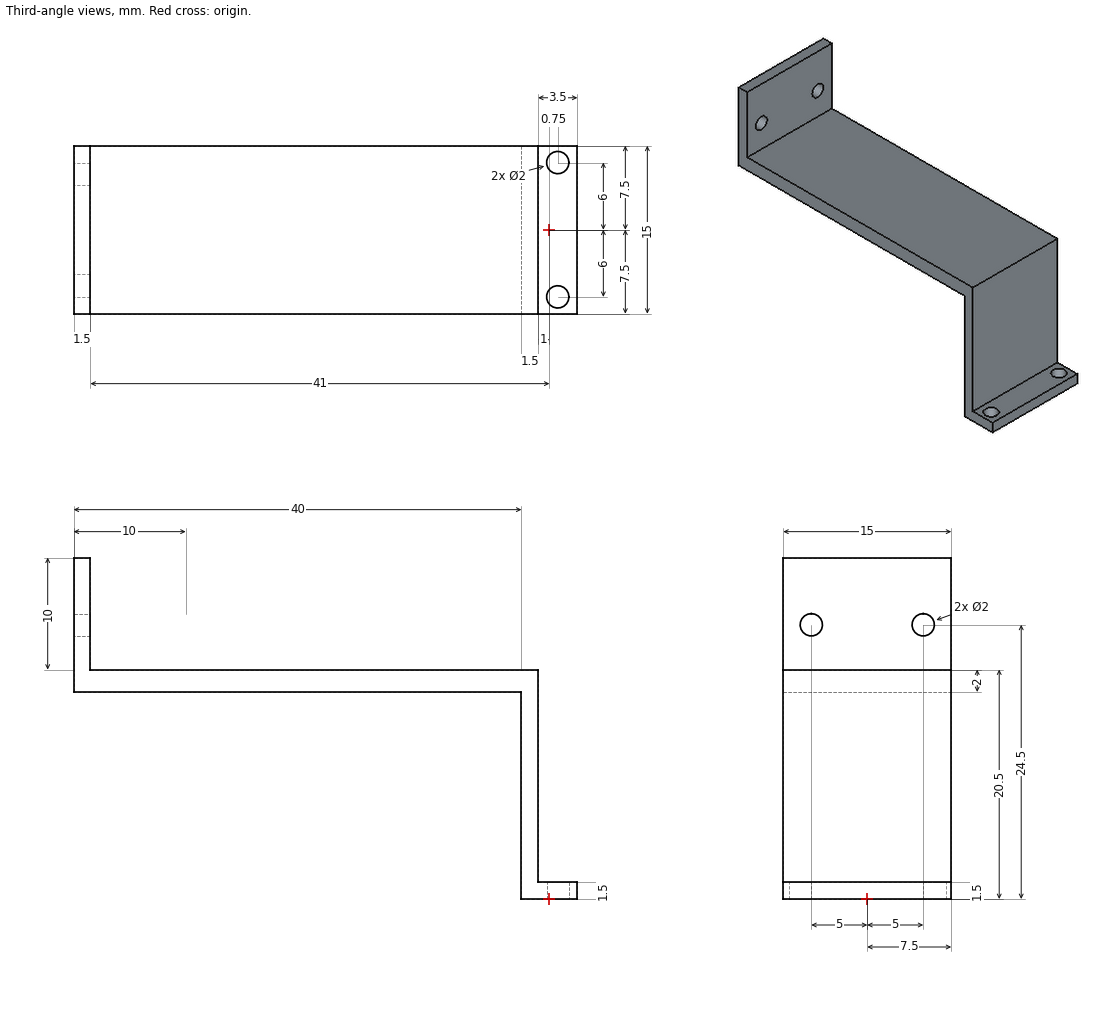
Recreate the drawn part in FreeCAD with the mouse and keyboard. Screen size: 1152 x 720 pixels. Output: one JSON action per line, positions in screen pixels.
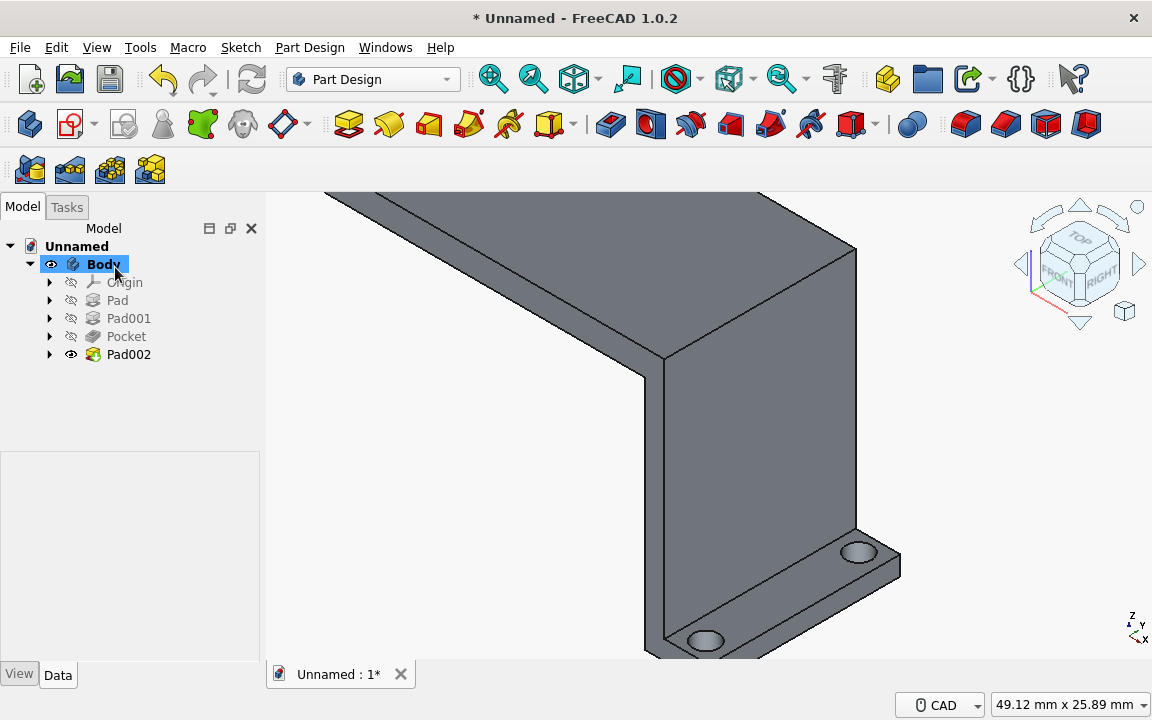
{"action": "left_click", "coordinate": [494, 80]}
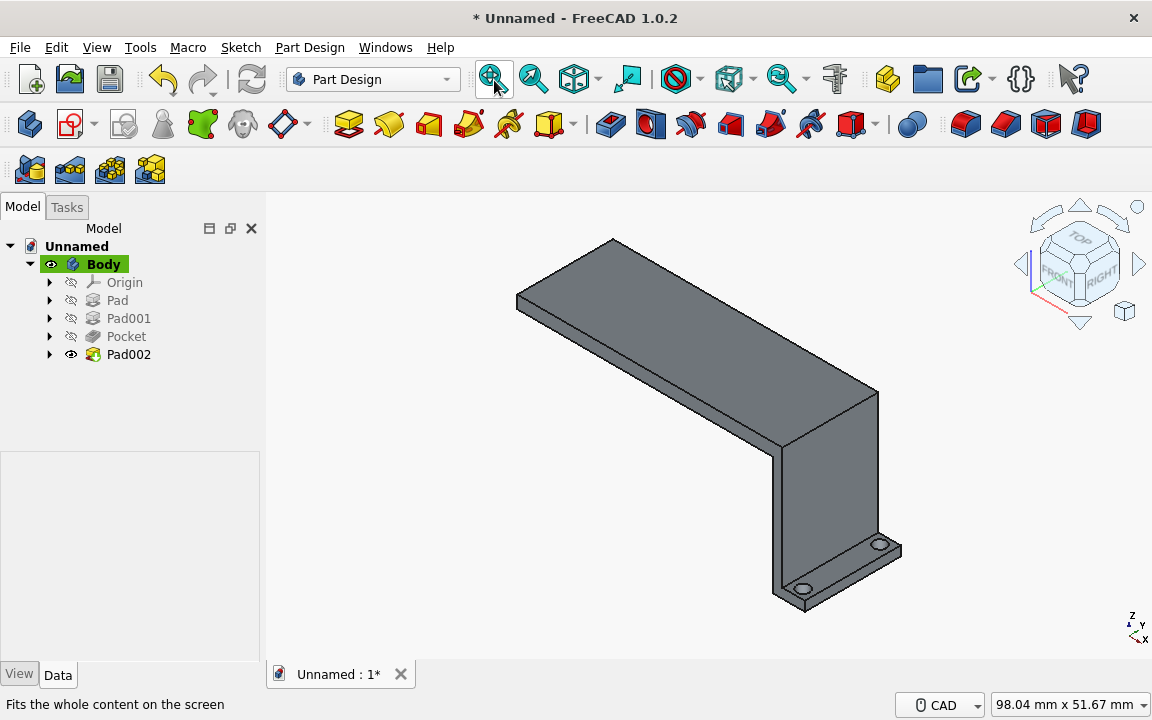
{"action": "left_click", "coordinate": [774, 386]}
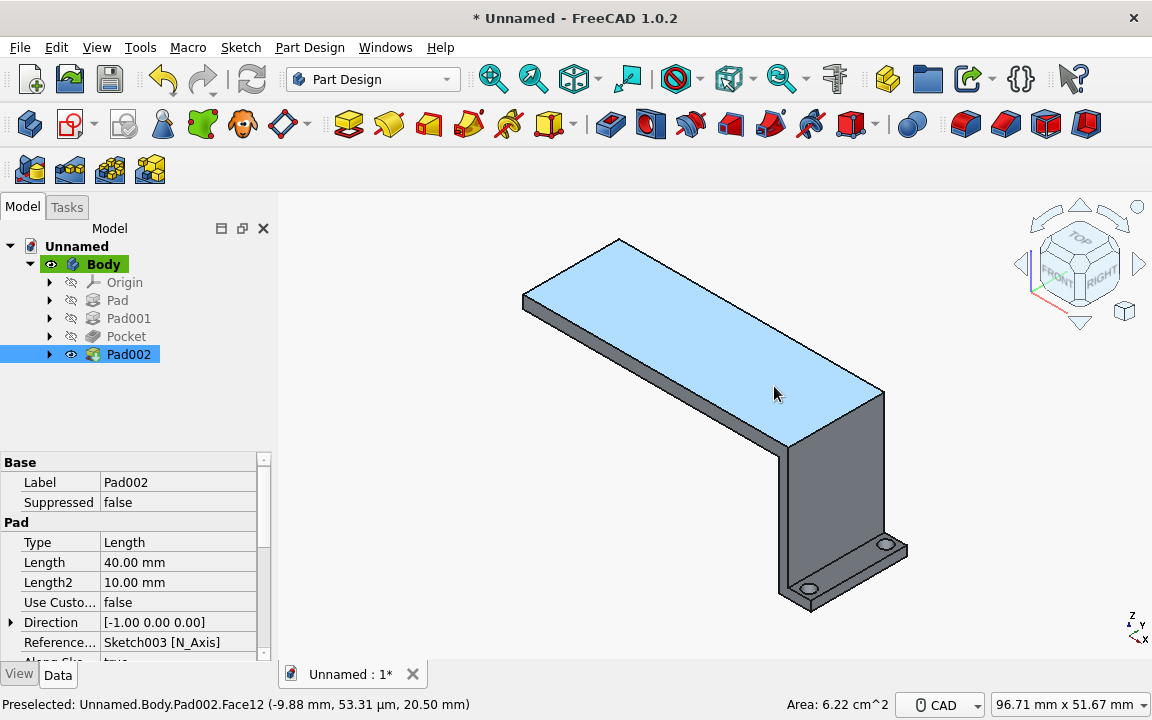
{"action": "left_click", "coordinate": [70, 124]}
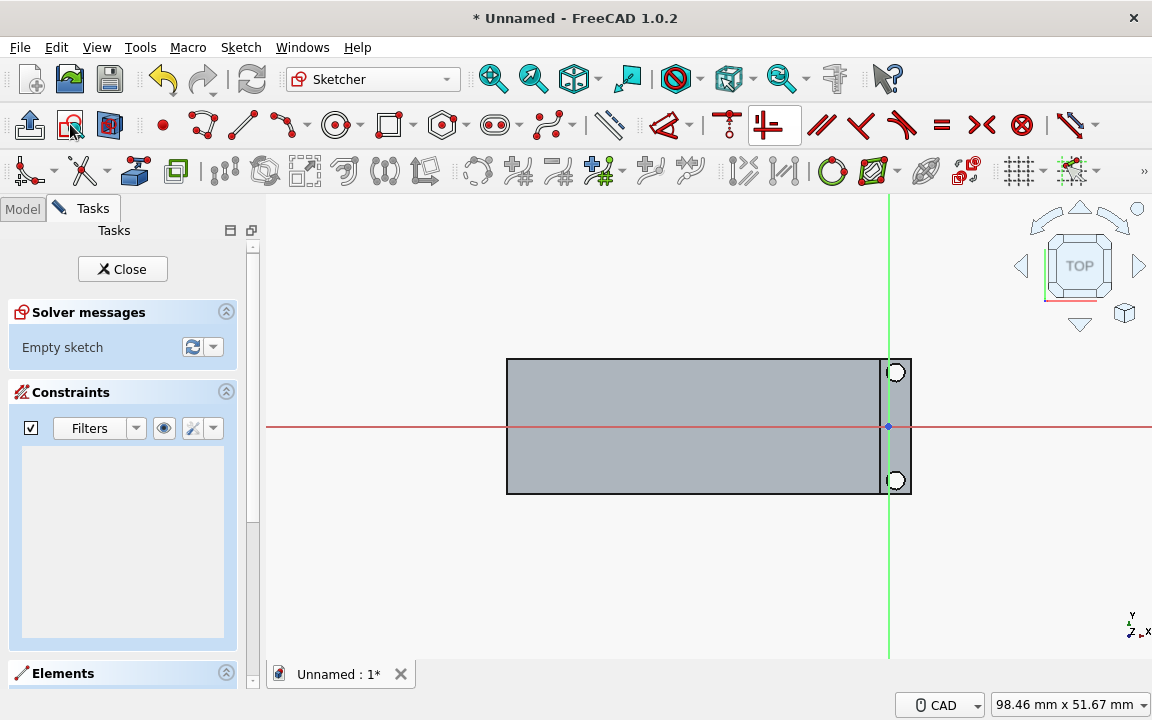
{"action": "scroll", "coordinate": [409, 426], "scroll_direction": "up", "scroll_amount": 4}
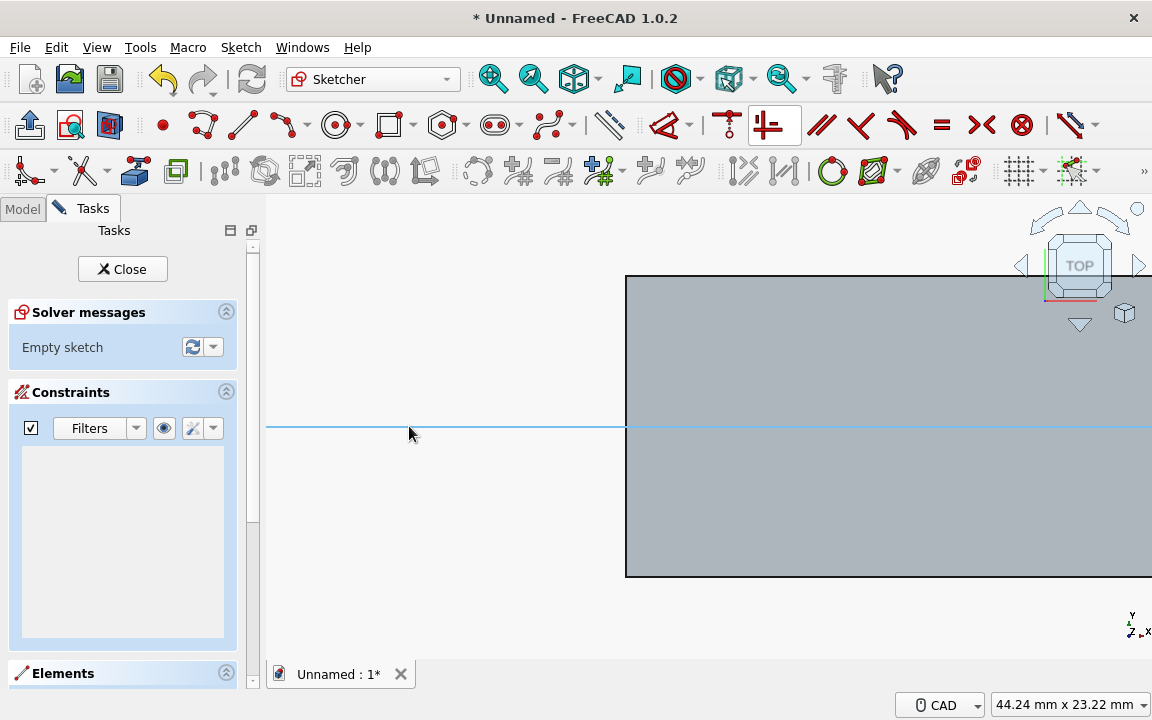
{"action": "left_click", "coordinate": [390, 126]}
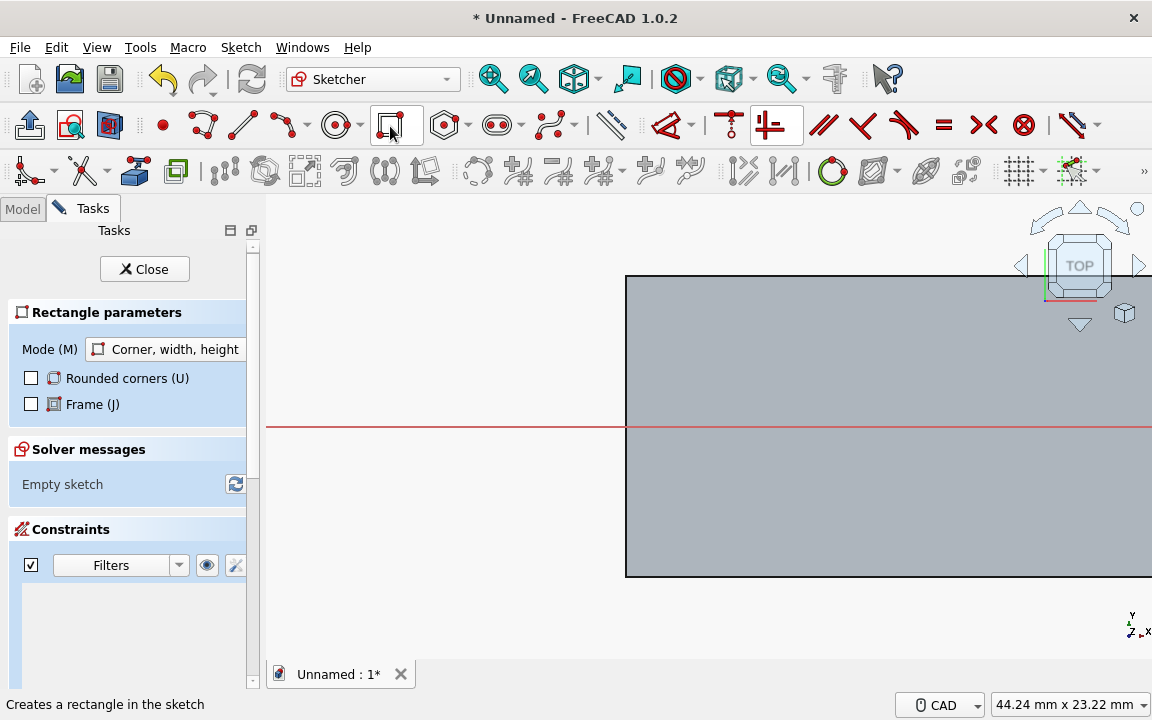
{"action": "left_click", "coordinate": [626, 276]}
{"action": "left_click", "coordinate": [656, 577]}
{"action": "key", "text": "Escape"}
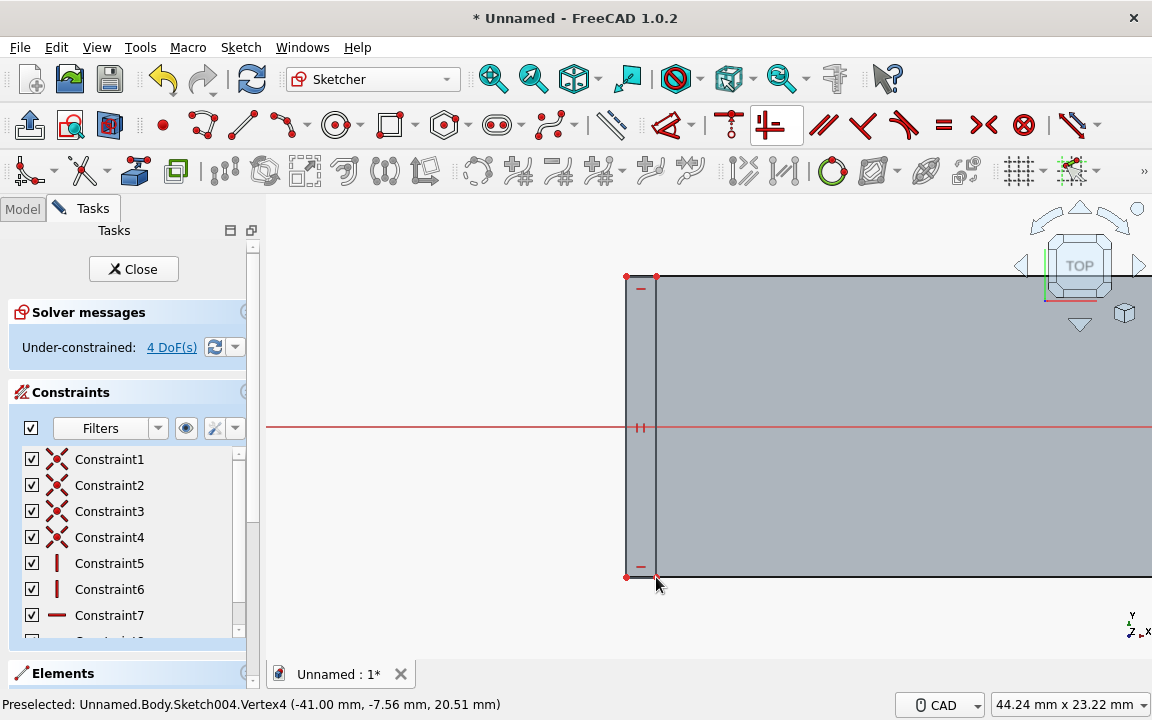
{"action": "left_click", "coordinate": [666, 126]}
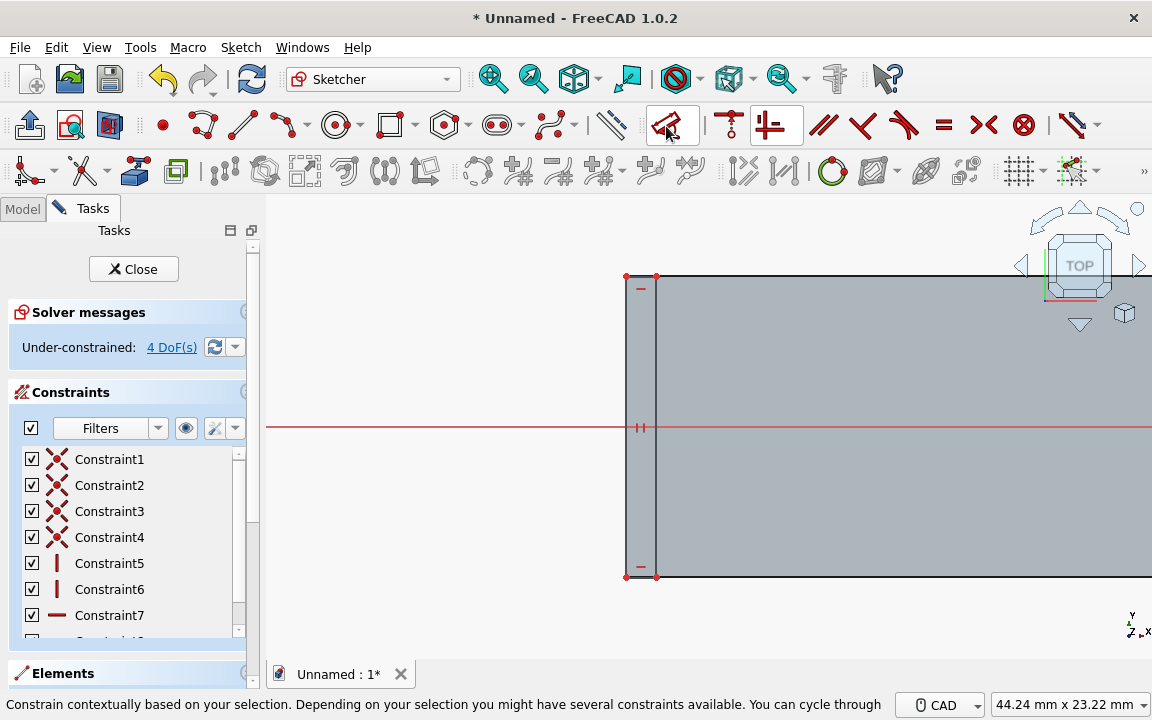
{"action": "left_click", "coordinate": [626, 367]}
{"action": "left_click", "coordinate": [592, 358]}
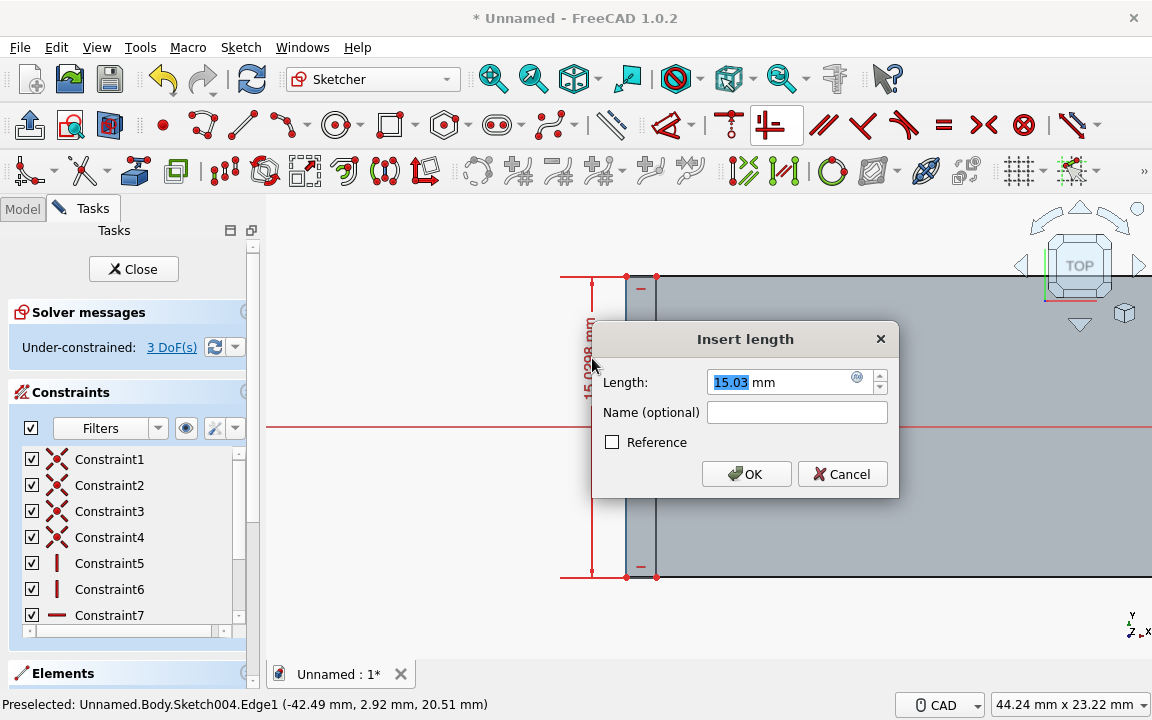
{"action": "type", "text": "15"}
{"action": "key", "text": "Return"}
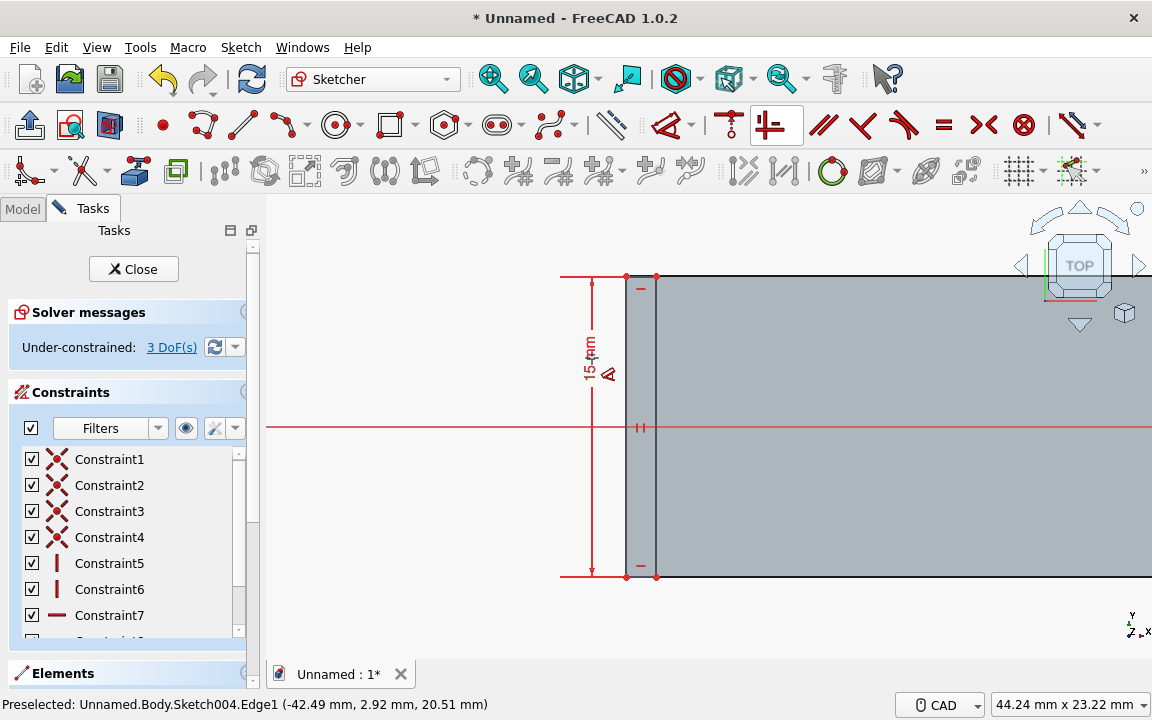
{"action": "scroll", "coordinate": [638, 577], "scroll_direction": "up", "scroll_amount": 2}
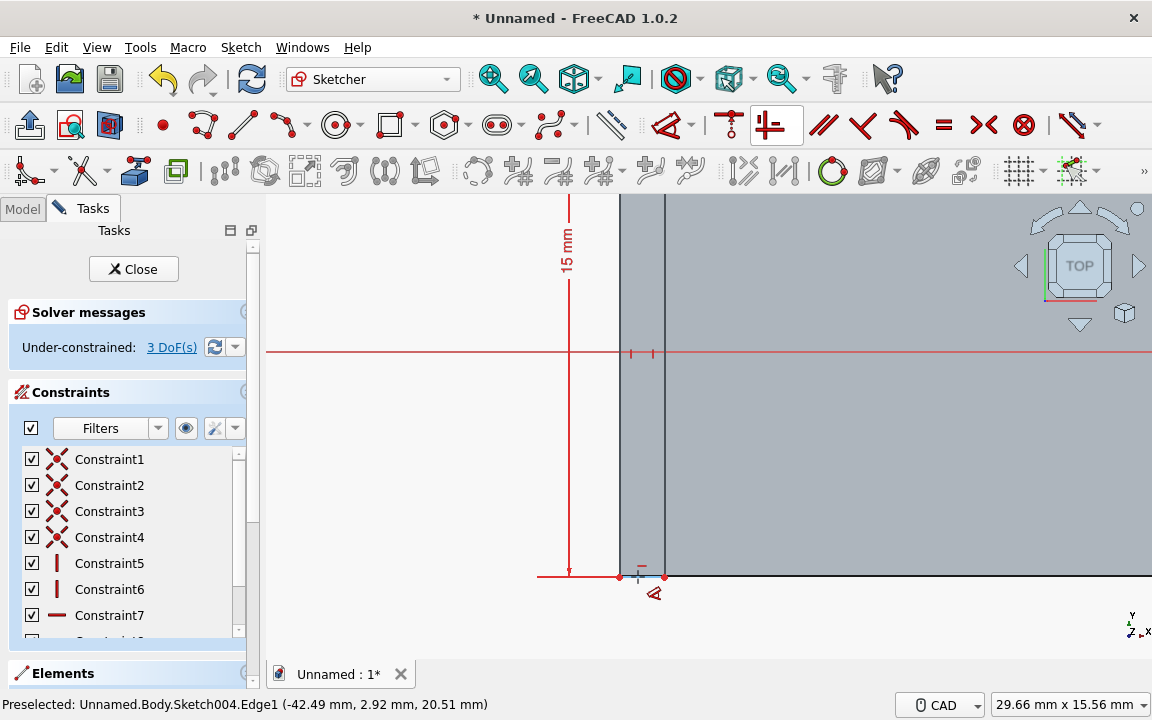
{"action": "left_click", "coordinate": [638, 577]}
{"action": "left_click", "coordinate": [642, 611]}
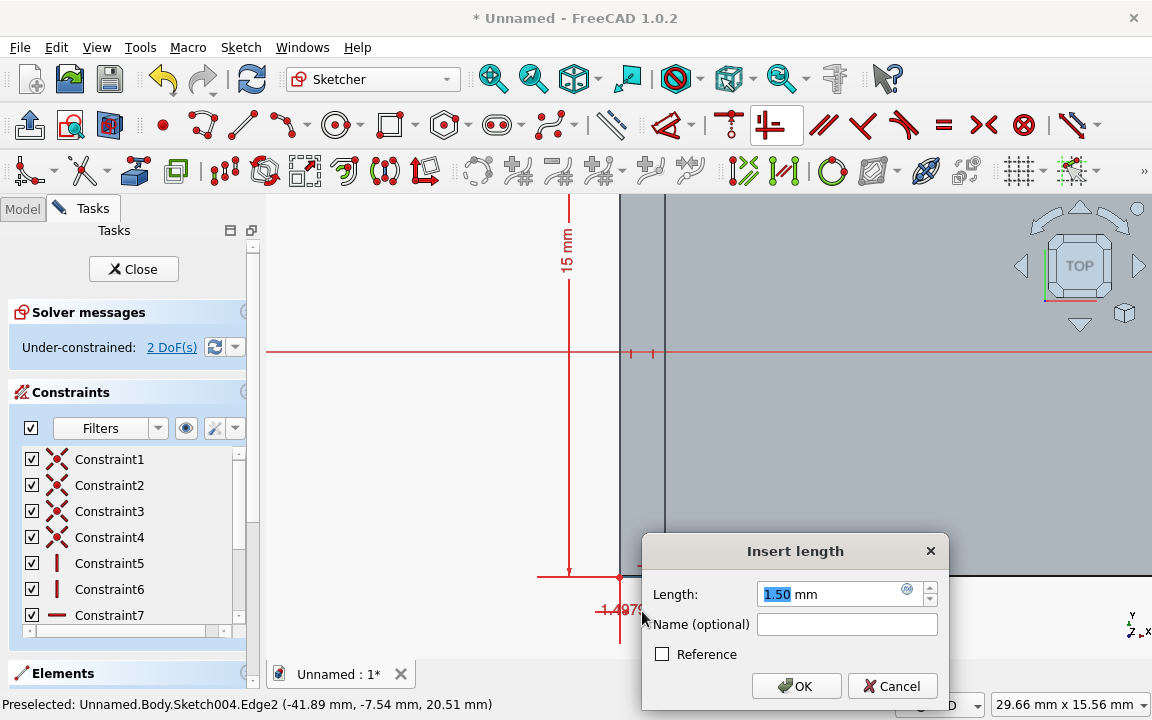
{"action": "type", "text": "1.5"}
{"action": "key", "text": "Return"}